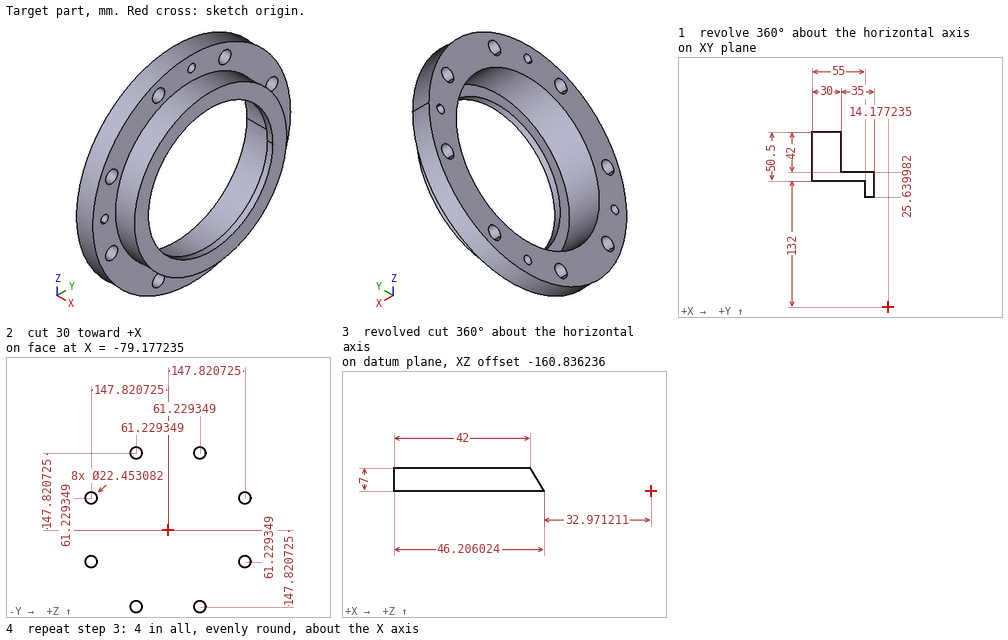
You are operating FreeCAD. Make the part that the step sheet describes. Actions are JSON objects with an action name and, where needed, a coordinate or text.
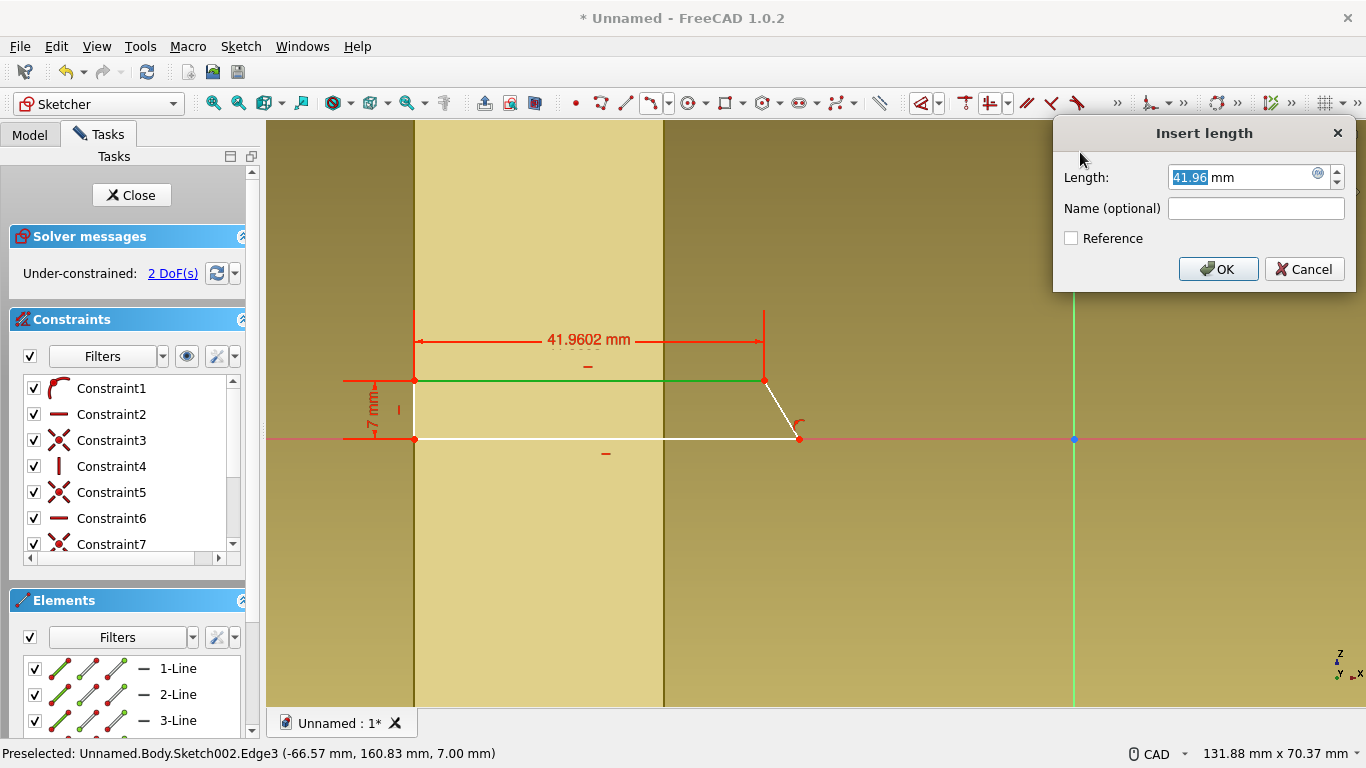
{"action": "type", "text": "42"}
{"action": "key", "text": "Return"}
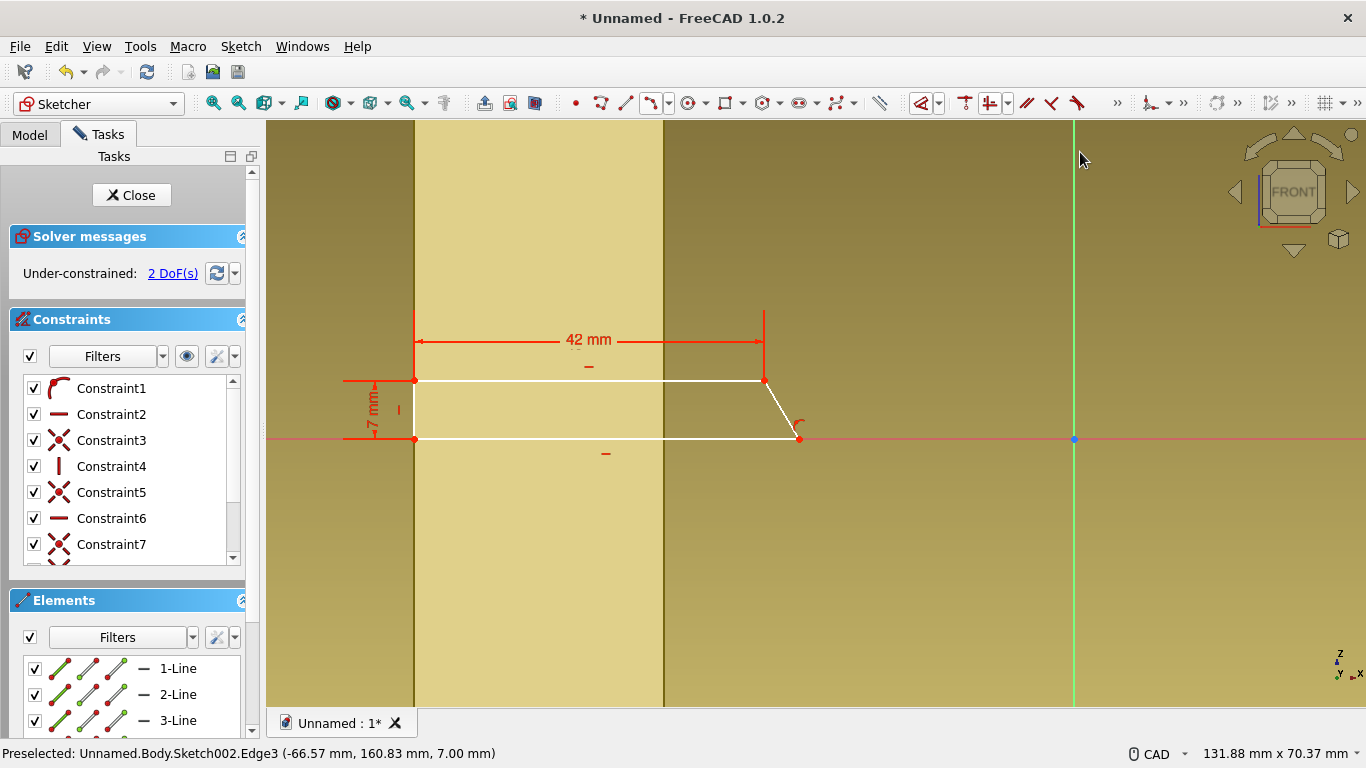
{"action": "left_click", "coordinate": [684, 439]}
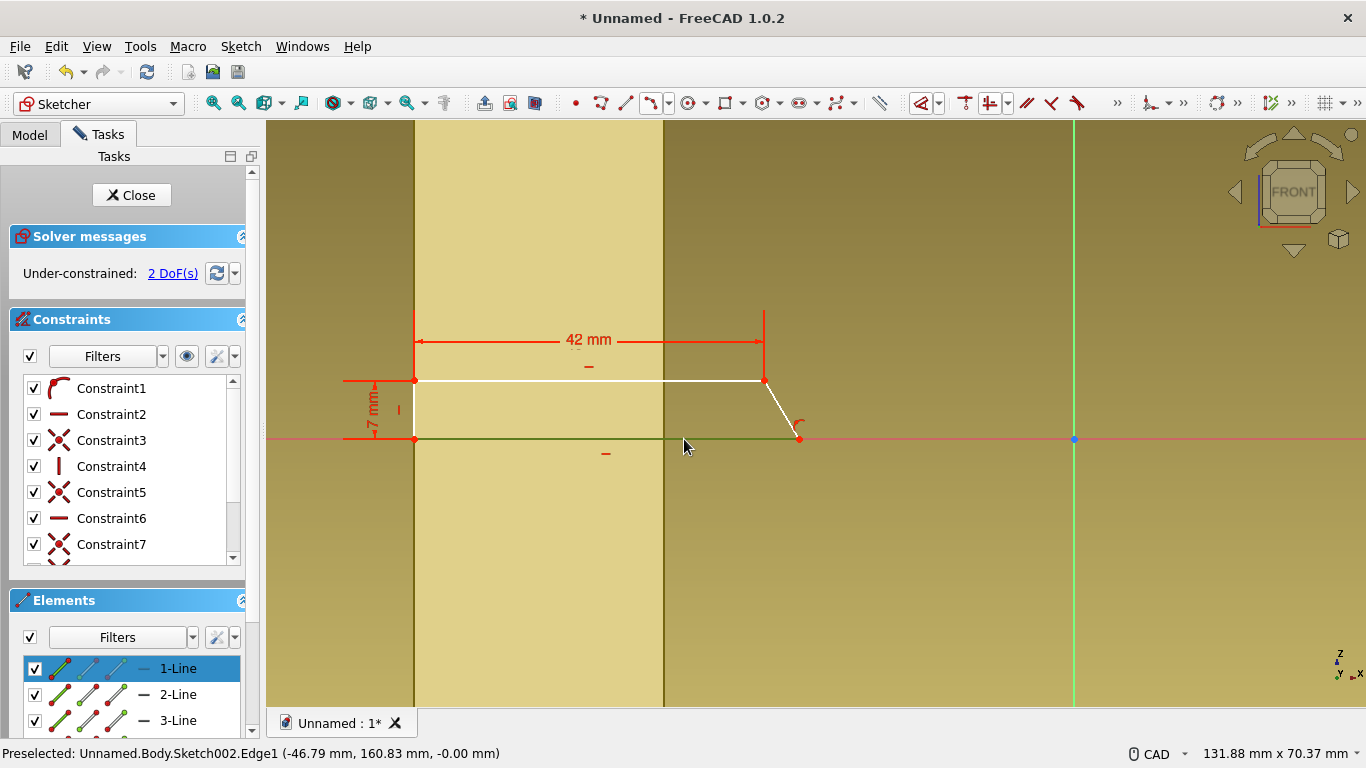
{"action": "left_click", "coordinate": [938, 104]}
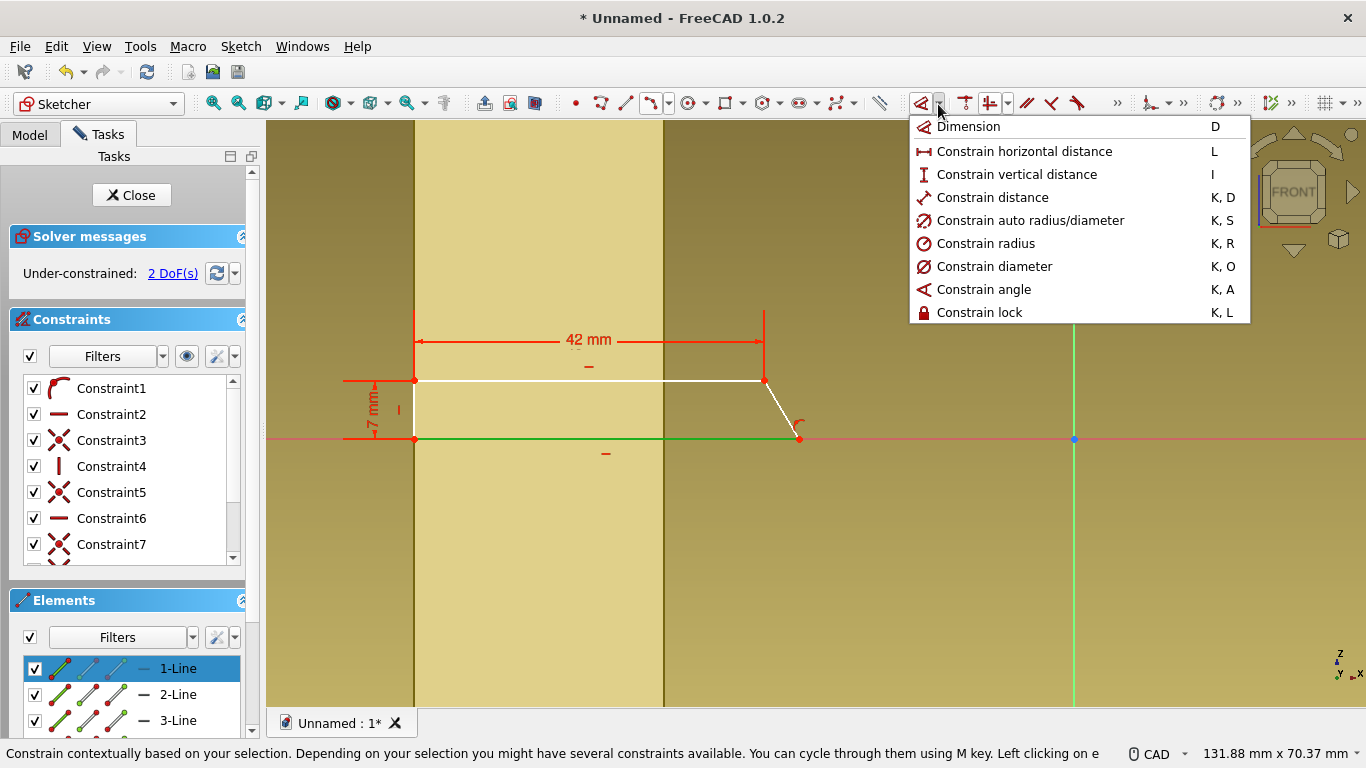
{"action": "left_click", "coordinate": [1080, 152]}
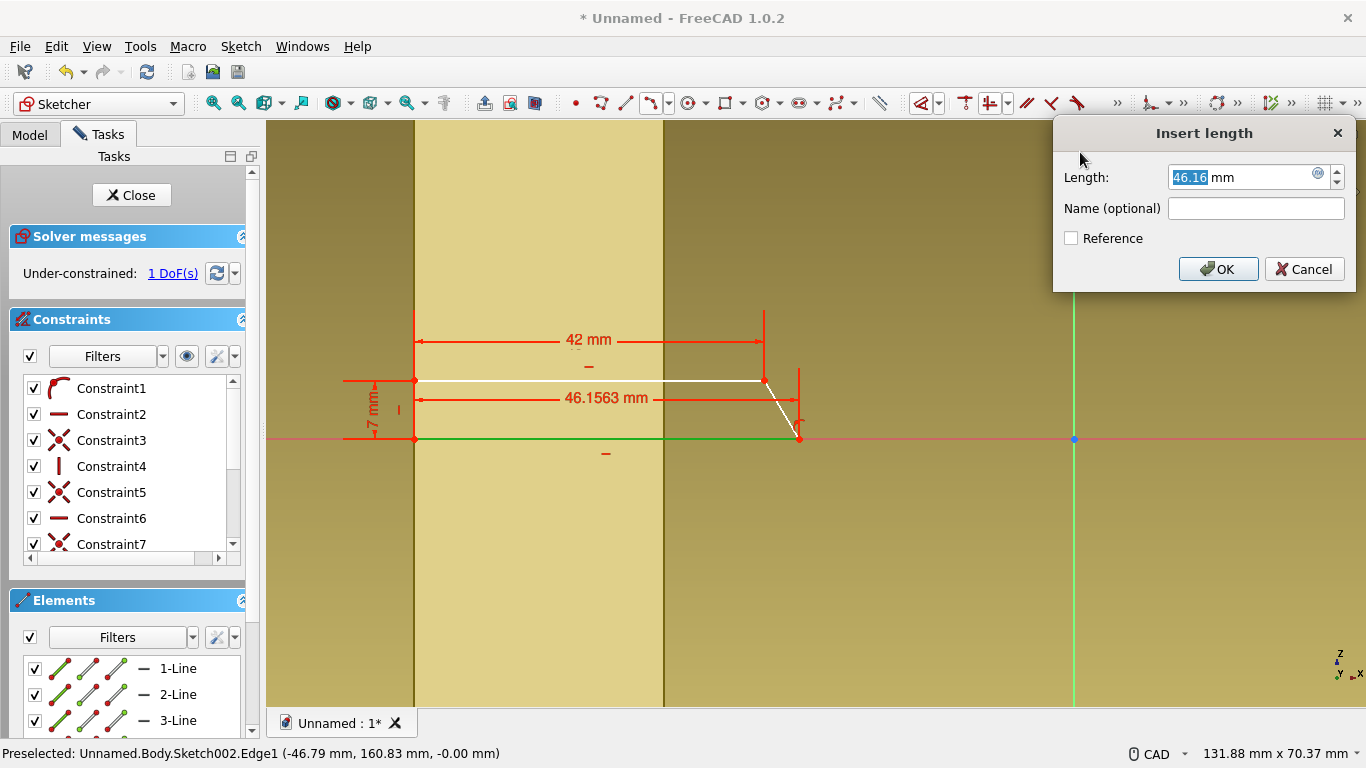
{"action": "type", "text": "46.206024"}
{"action": "key", "text": "Return"}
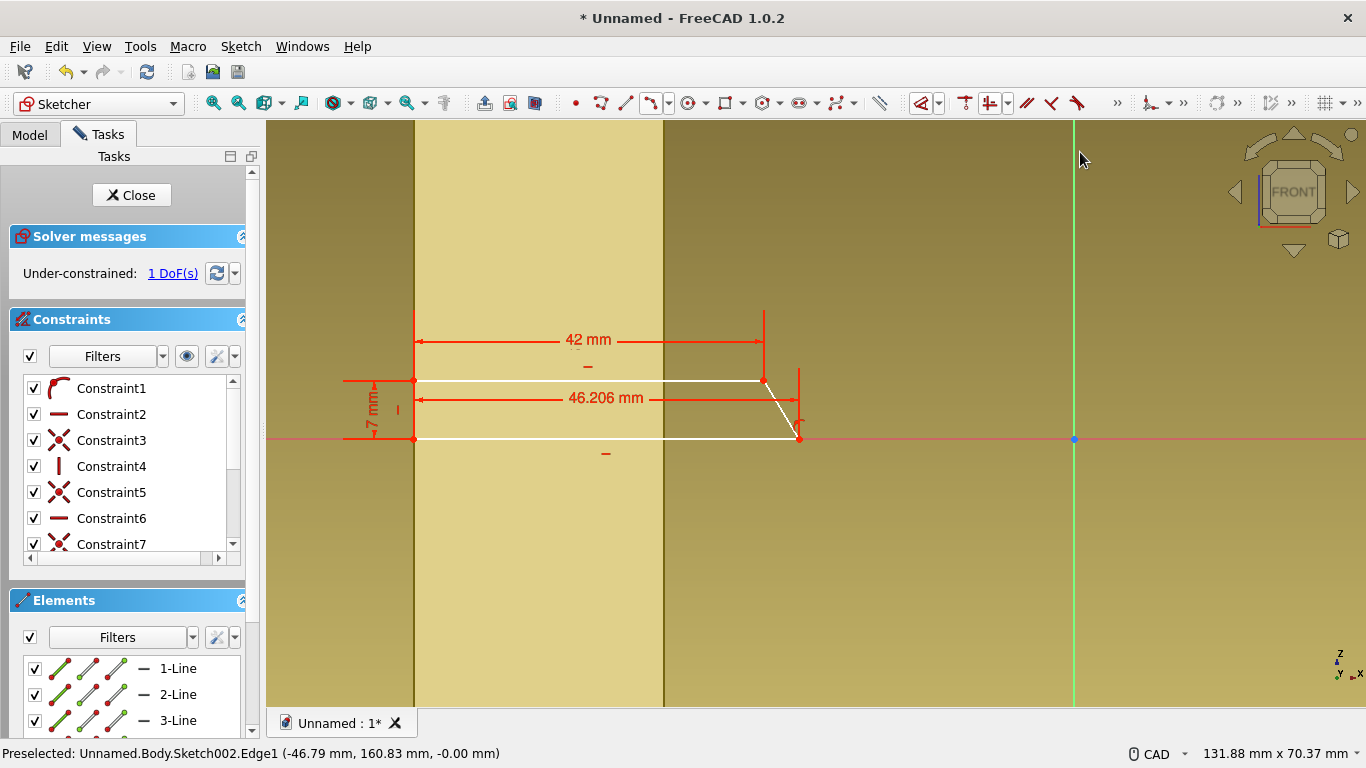
{"action": "left_click", "coordinate": [799, 439]}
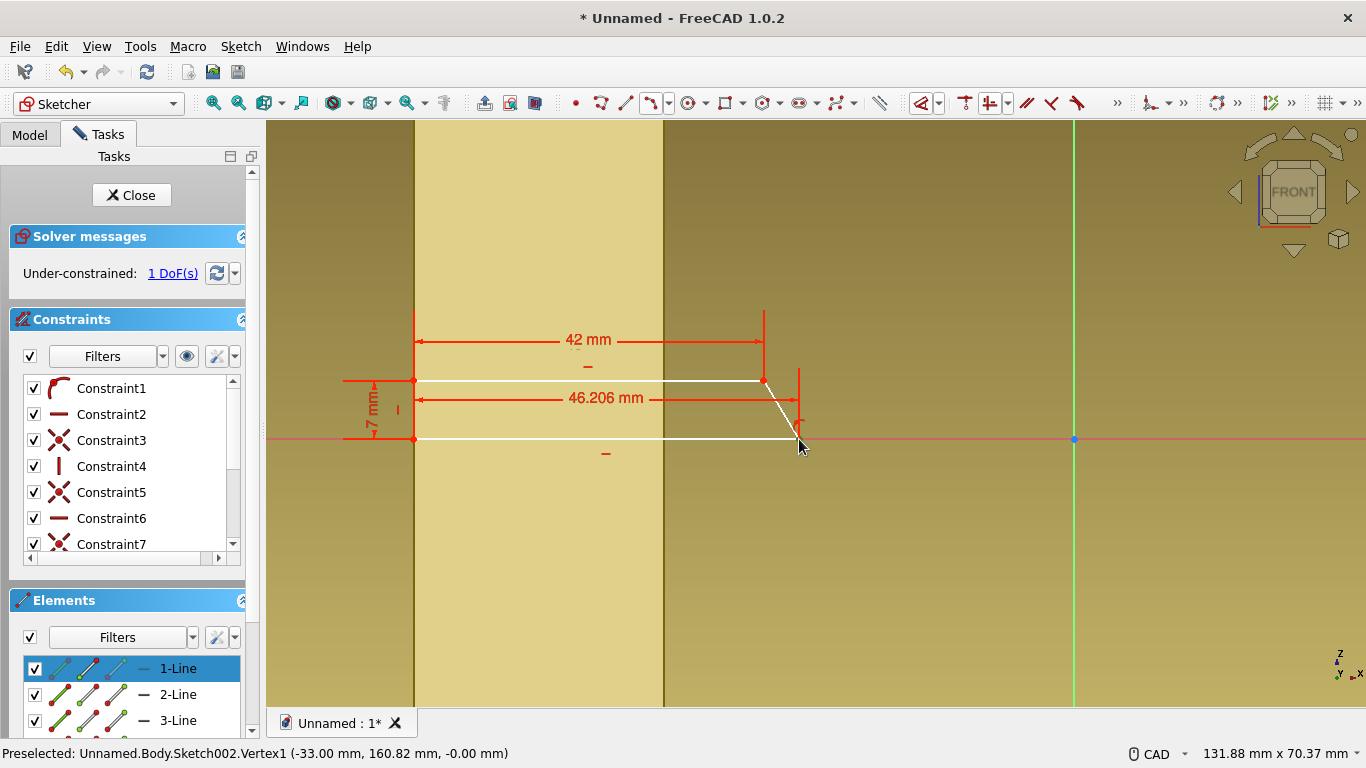
{"action": "key", "text": "l"}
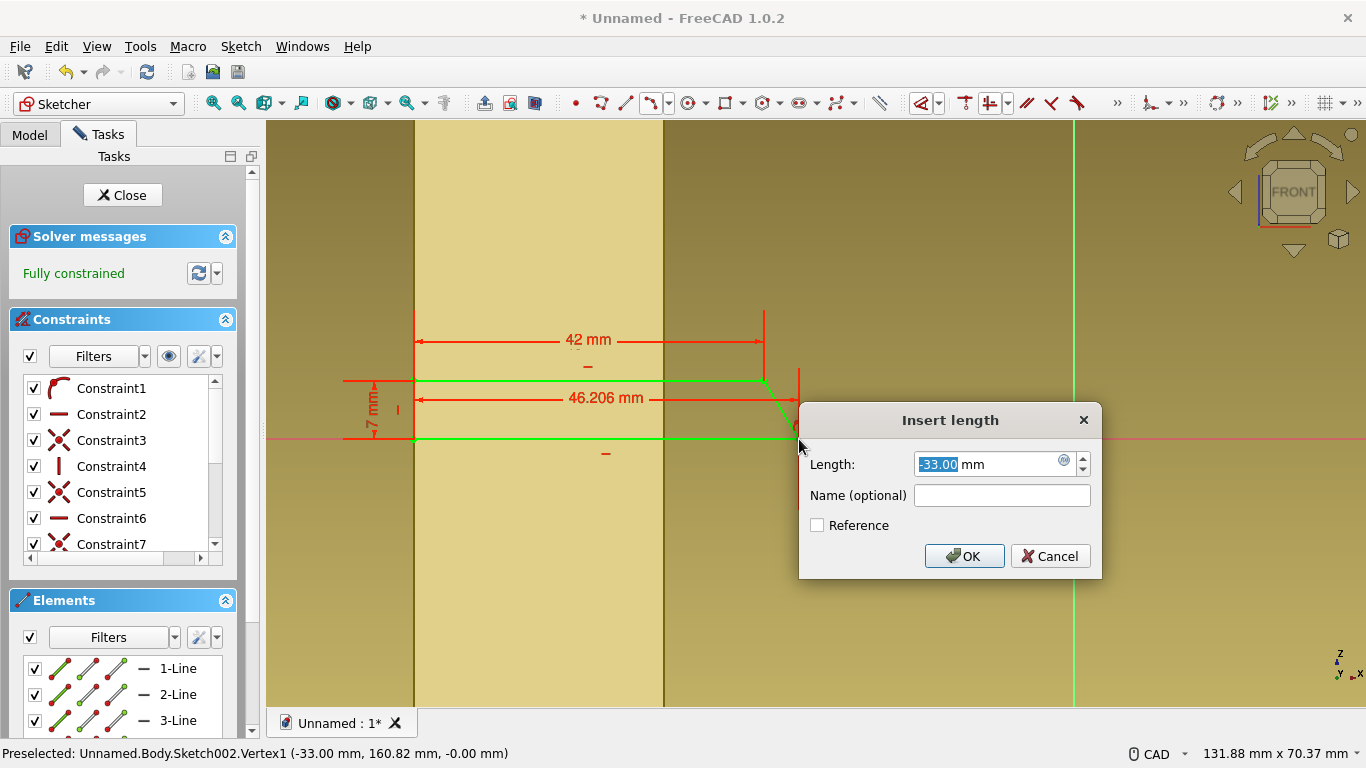
{"action": "type", "text": "-32.971211"}
{"action": "key", "text": "Return"}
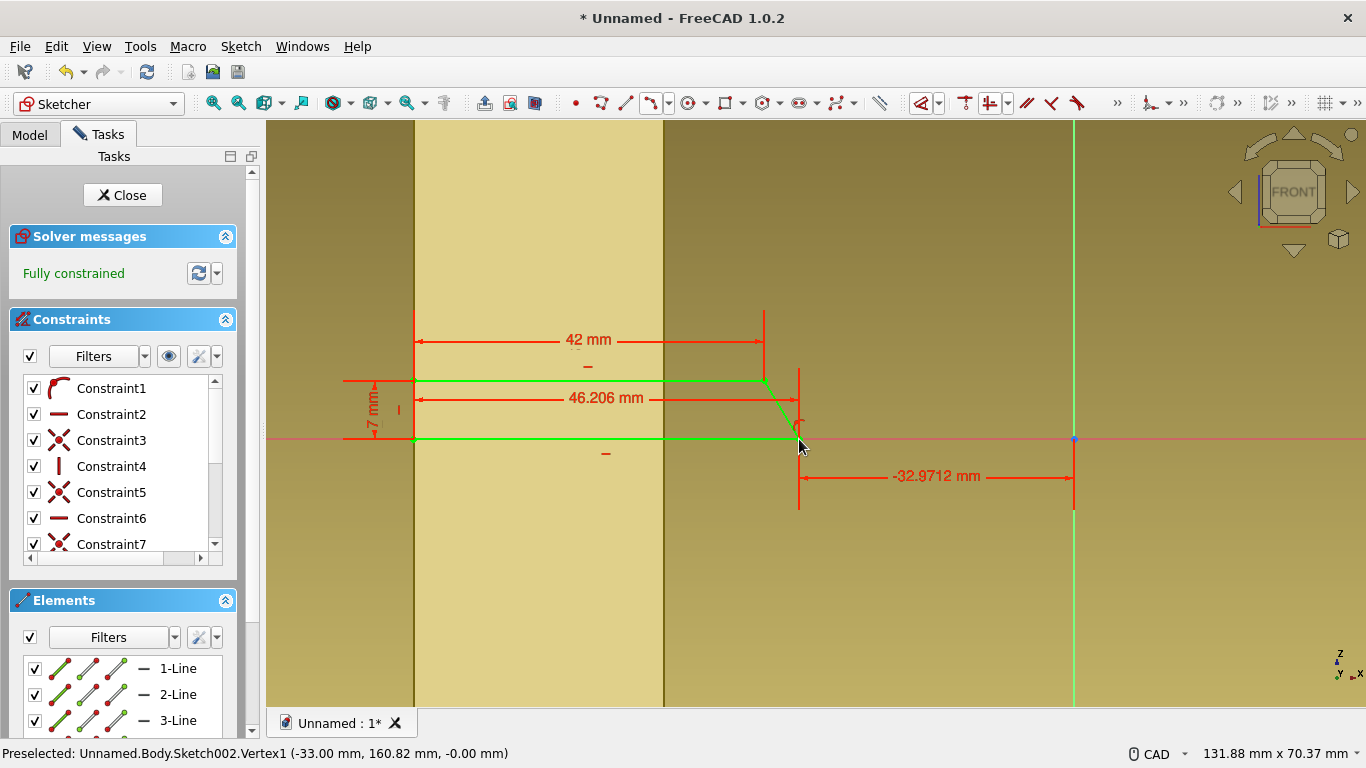
{"action": "left_click", "coordinate": [123, 195]}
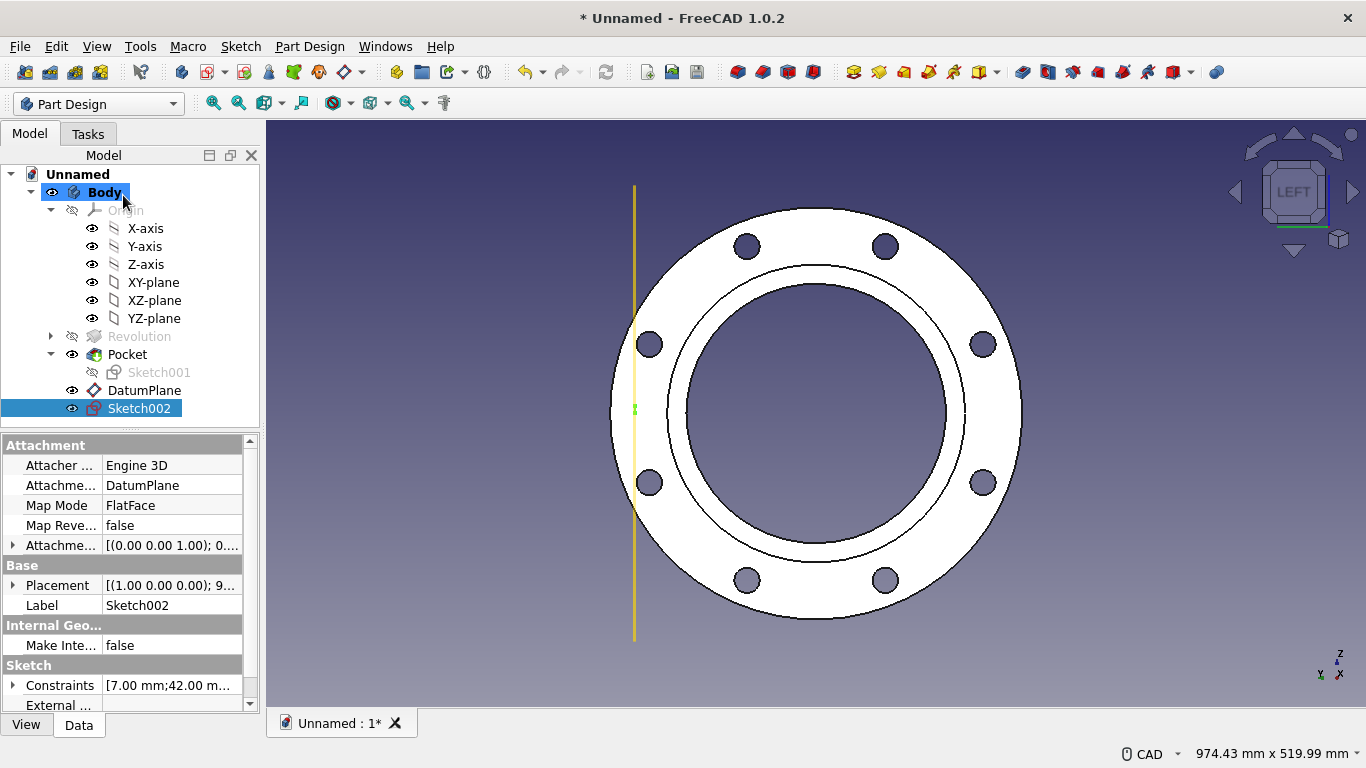
{"action": "left_click", "coordinate": [1073, 72]}